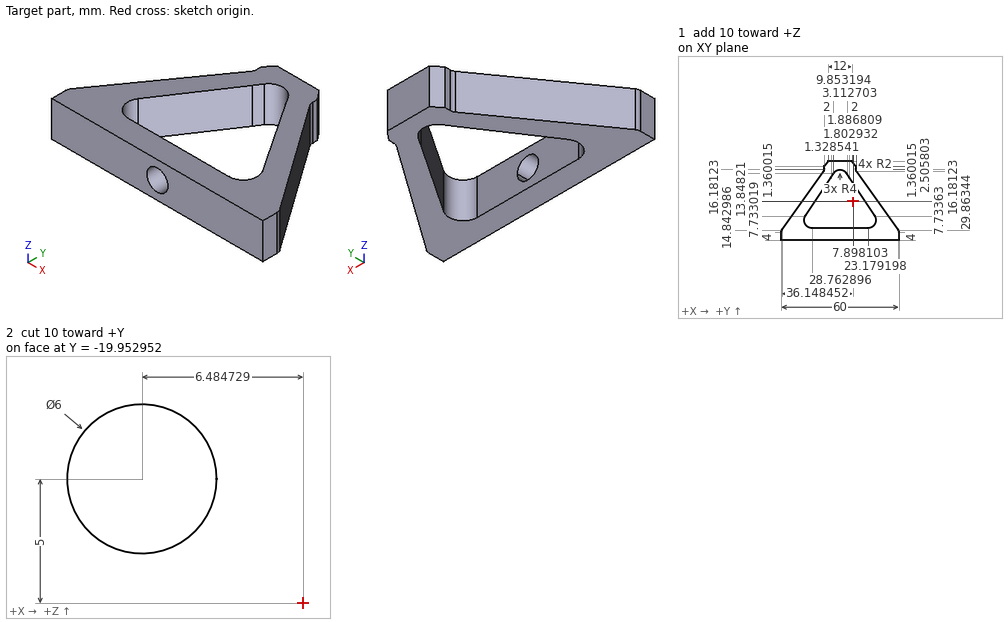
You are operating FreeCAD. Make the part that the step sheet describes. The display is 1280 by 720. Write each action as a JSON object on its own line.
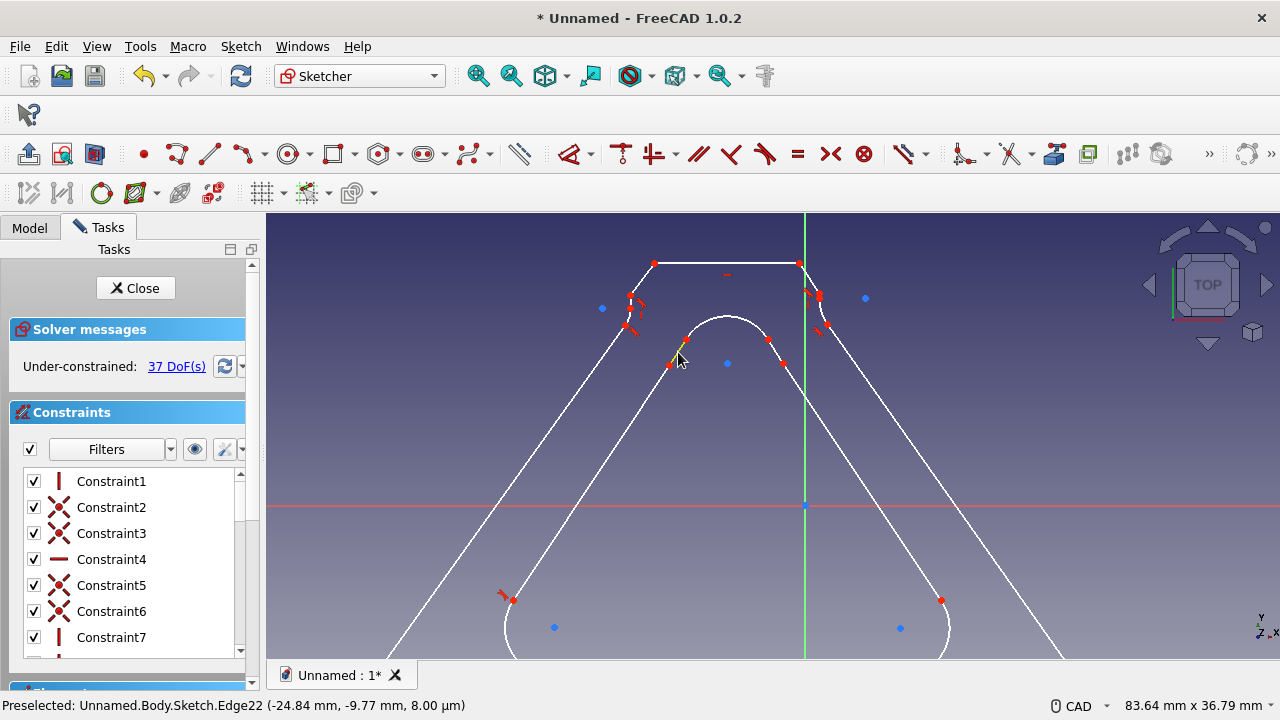
{"action": "left_click", "coordinate": [678, 352]}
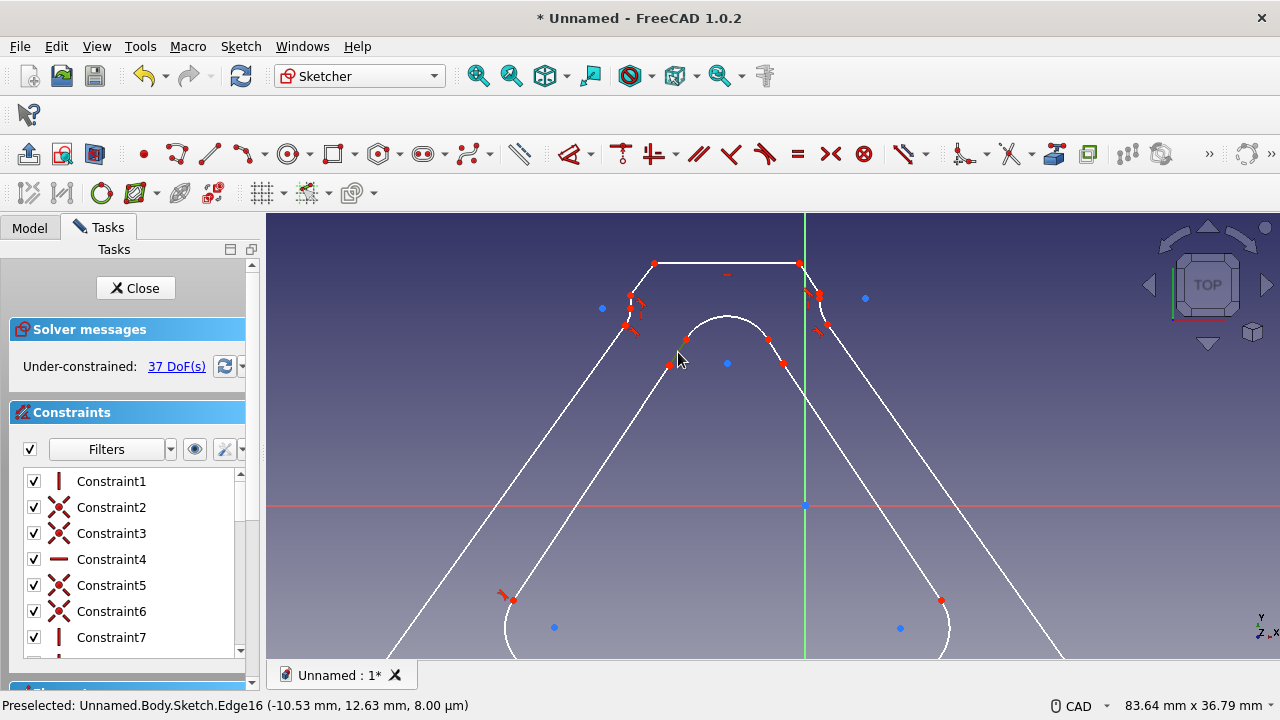
{"action": "left_click", "coordinate": [746, 320]}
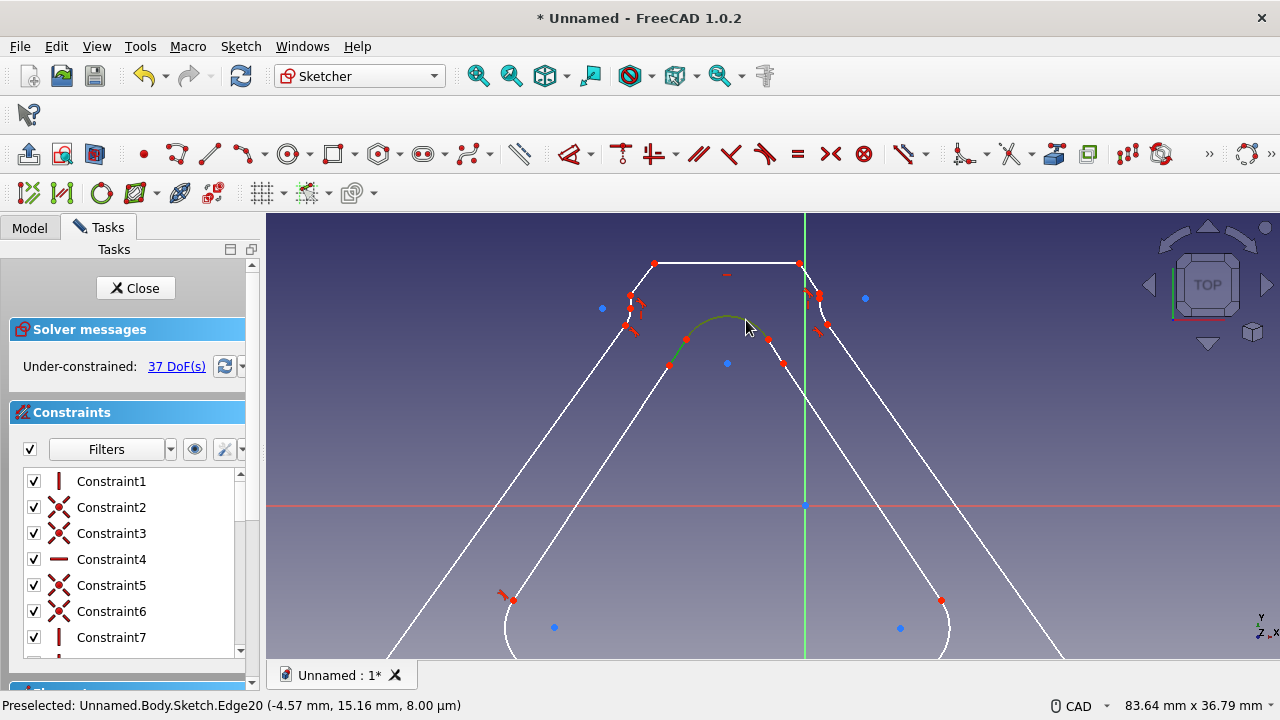
{"action": "left_click", "coordinate": [765, 154]}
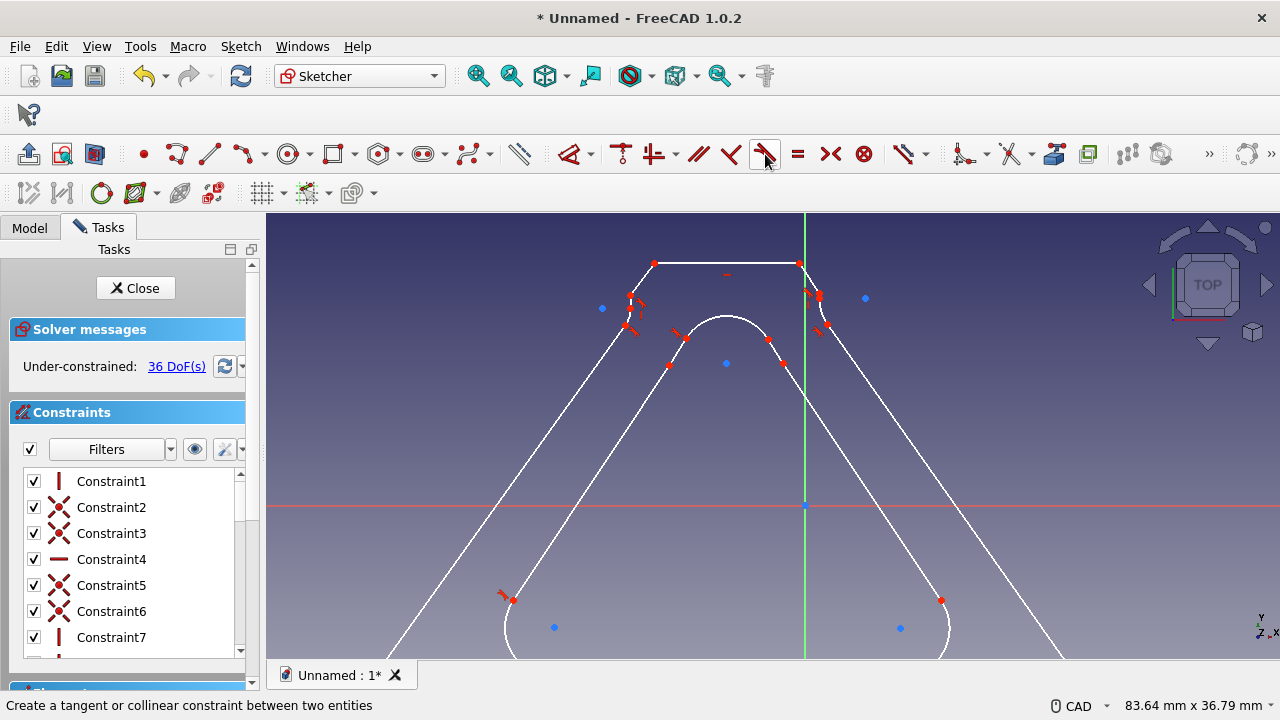
{"action": "scroll", "coordinate": [774, 349], "scroll_direction": "up", "scroll_amount": 2}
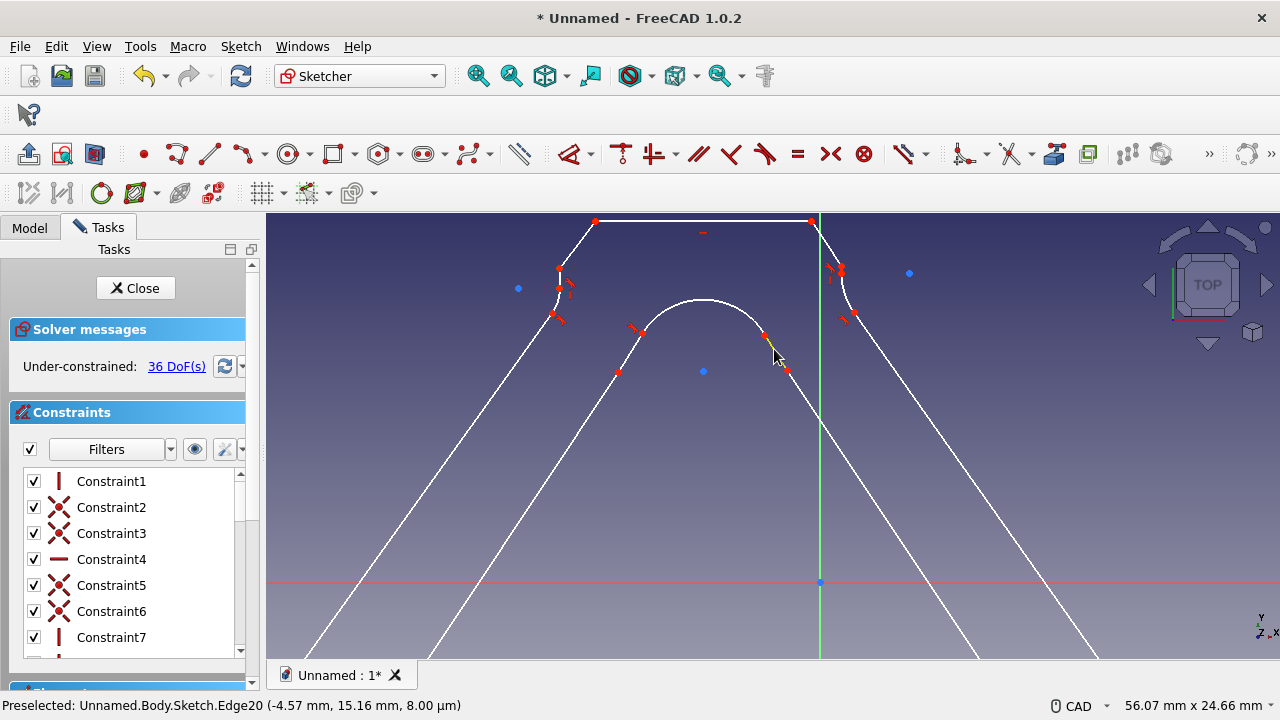
{"action": "left_click", "coordinate": [774, 349]}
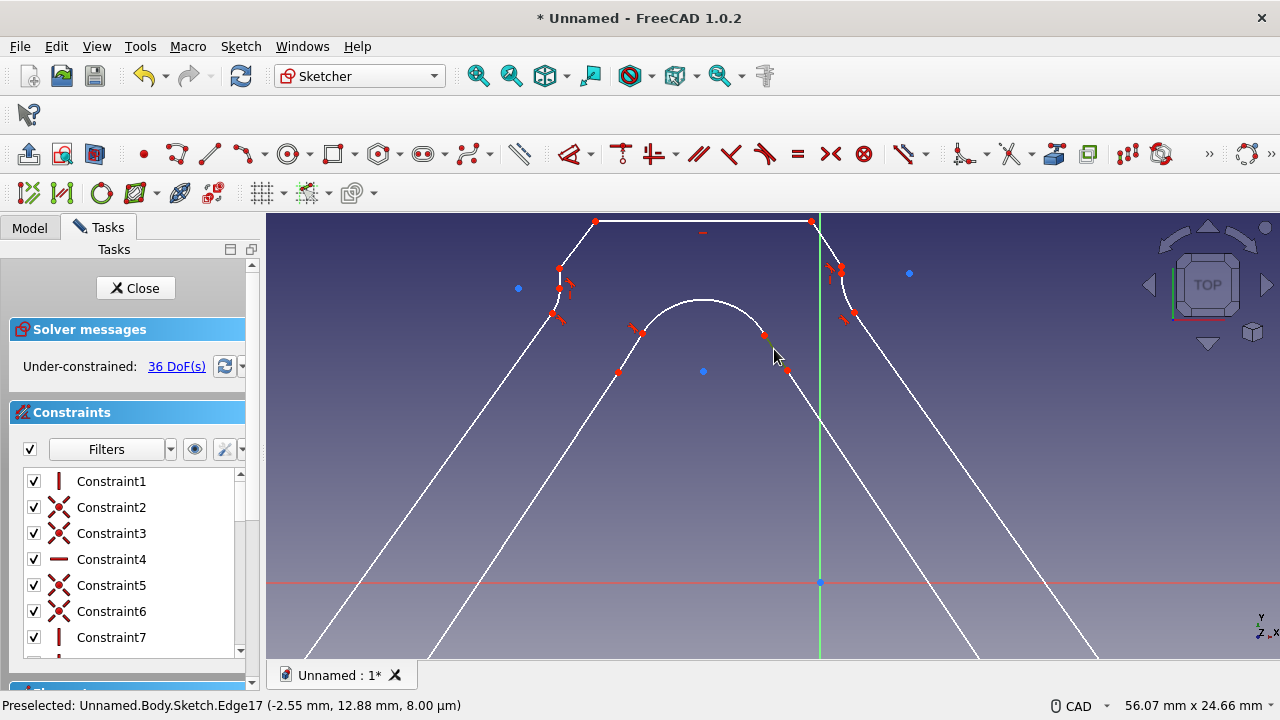
{"action": "left_click", "coordinate": [733, 306]}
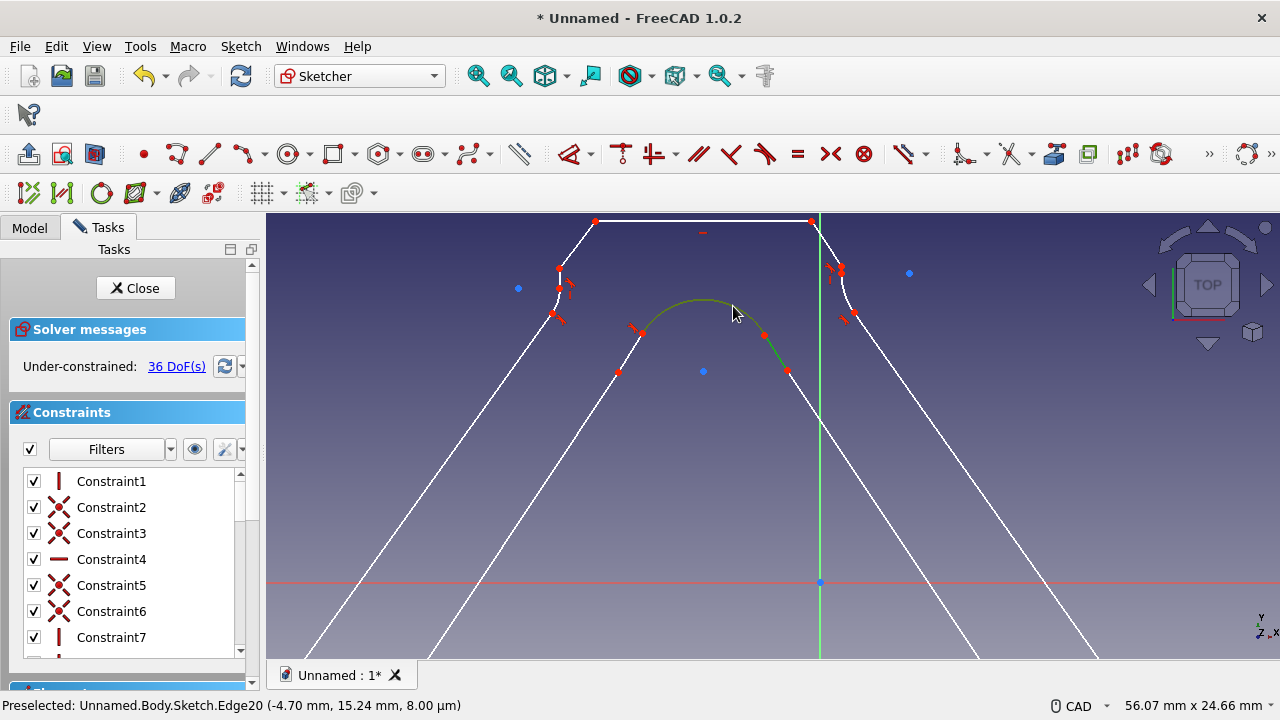
{"action": "left_click", "coordinate": [765, 154]}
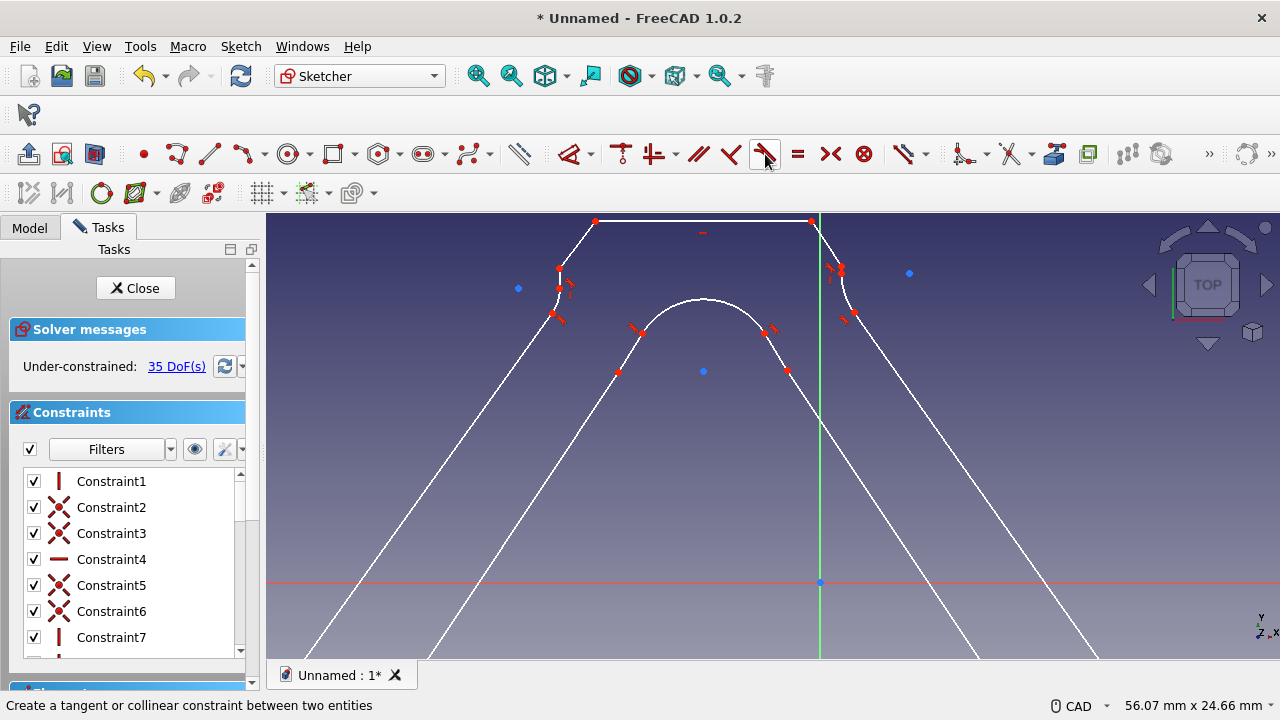
{"action": "left_click", "coordinate": [858, 477]}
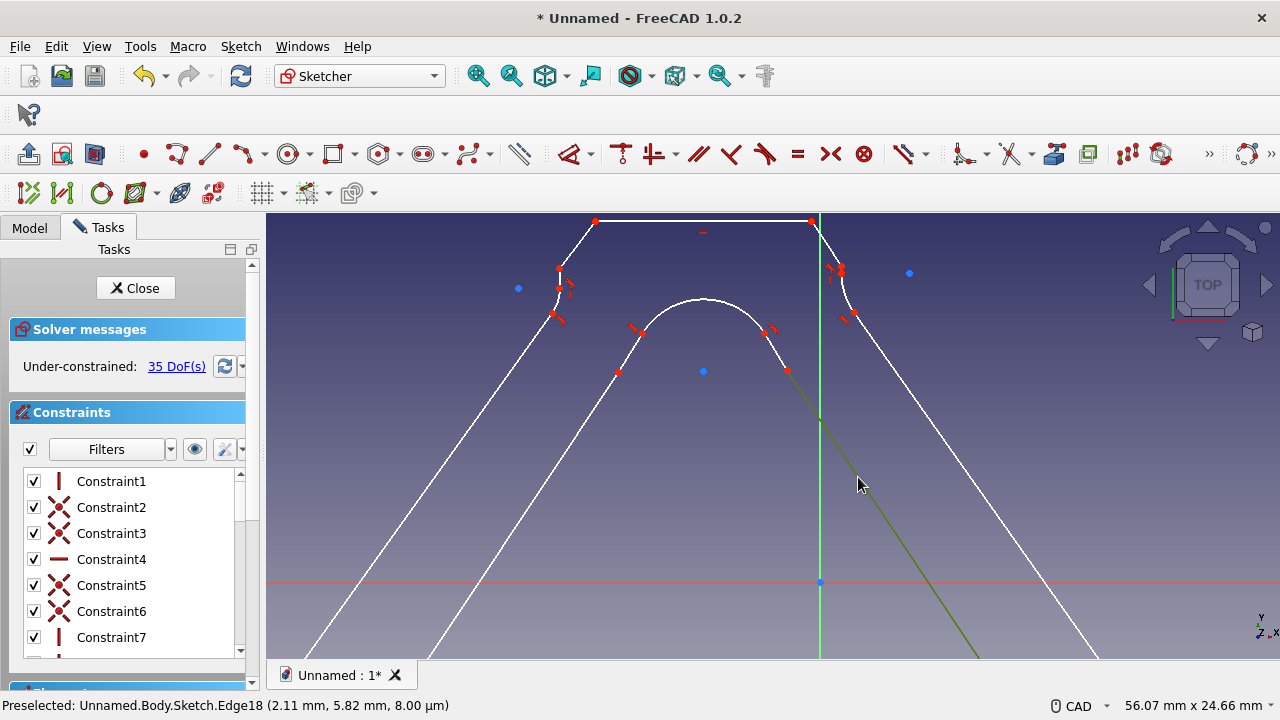
{"action": "scroll", "coordinate": [705, 351], "scroll_direction": "down", "scroll_amount": 5}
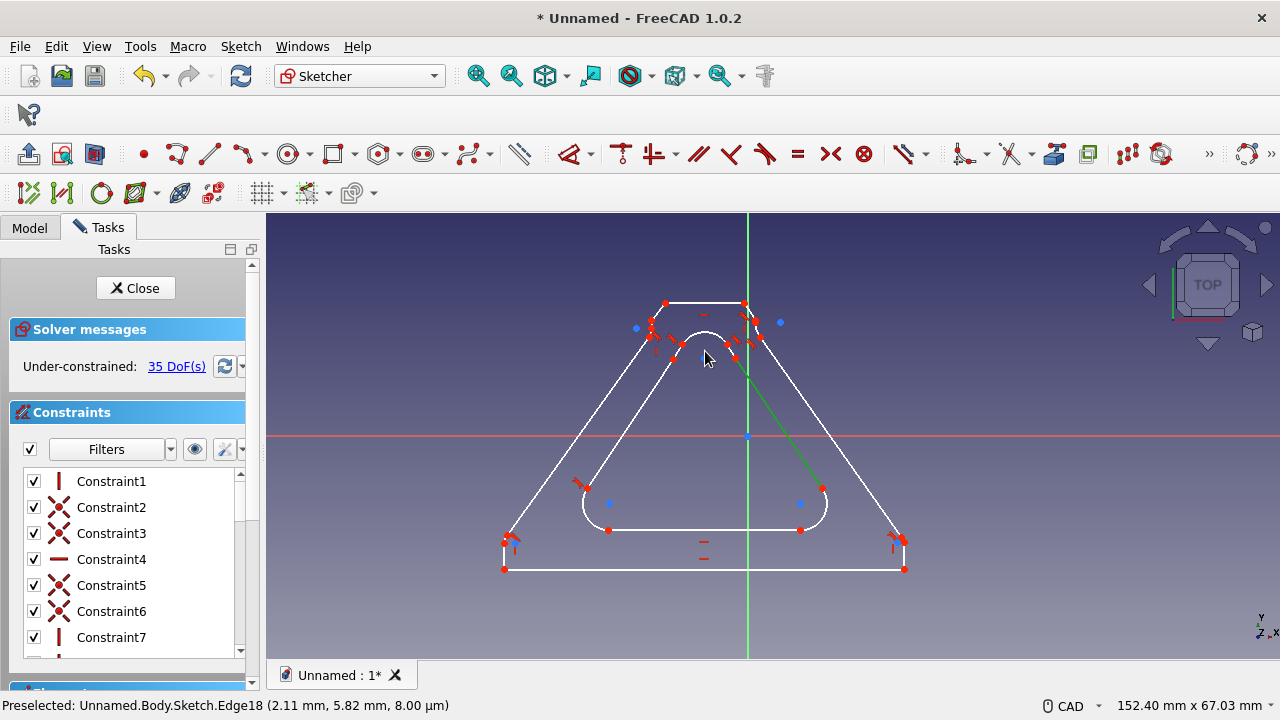
{"action": "left_click", "coordinate": [816, 525]}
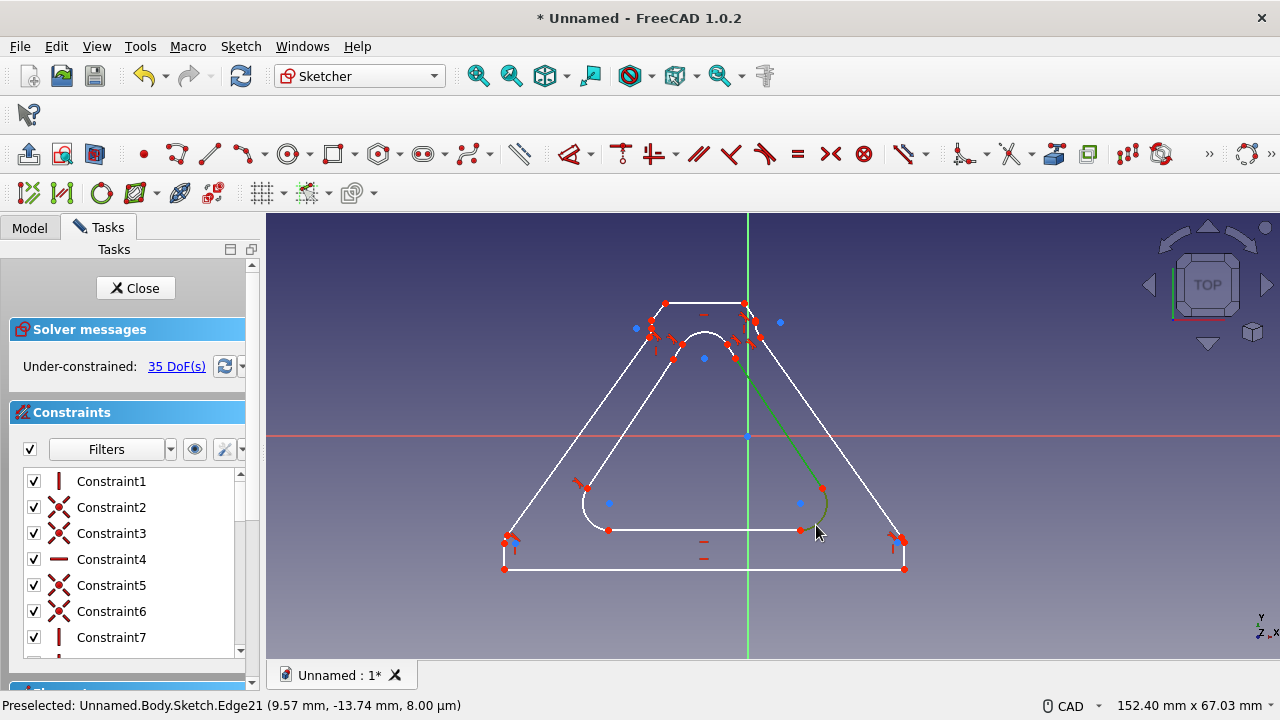
{"action": "left_click", "coordinate": [765, 154]}